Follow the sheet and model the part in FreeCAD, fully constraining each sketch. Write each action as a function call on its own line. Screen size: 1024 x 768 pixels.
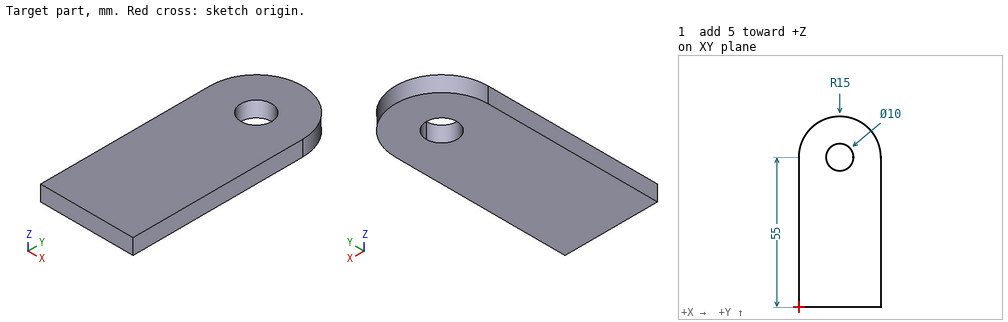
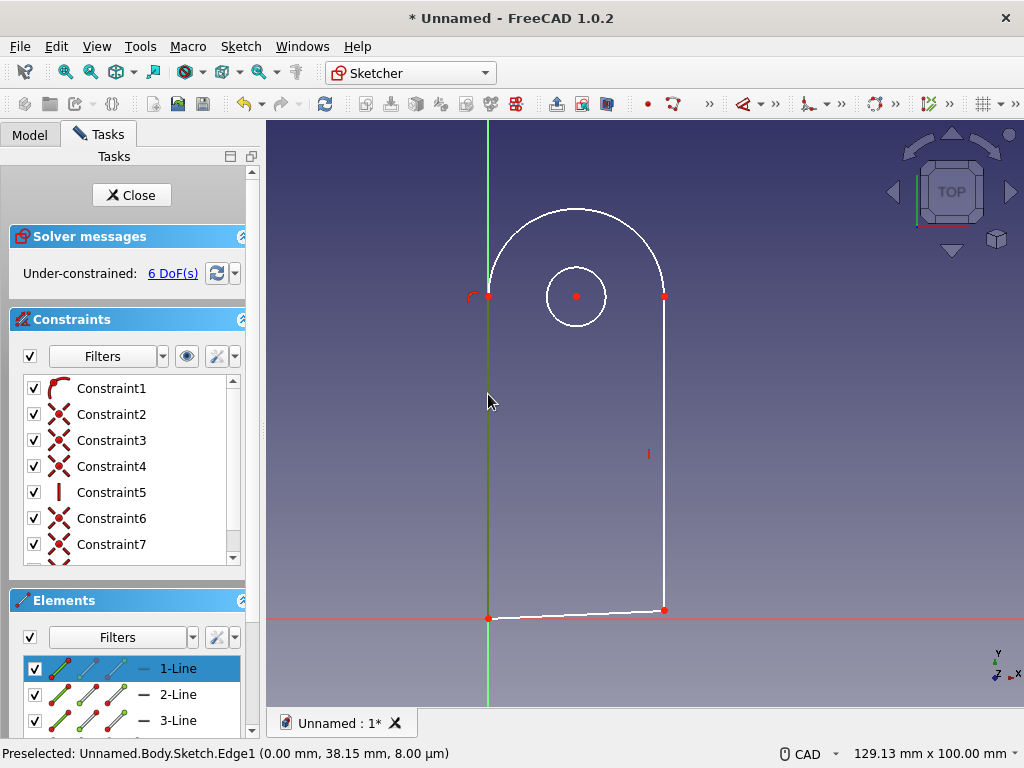
click(628, 226)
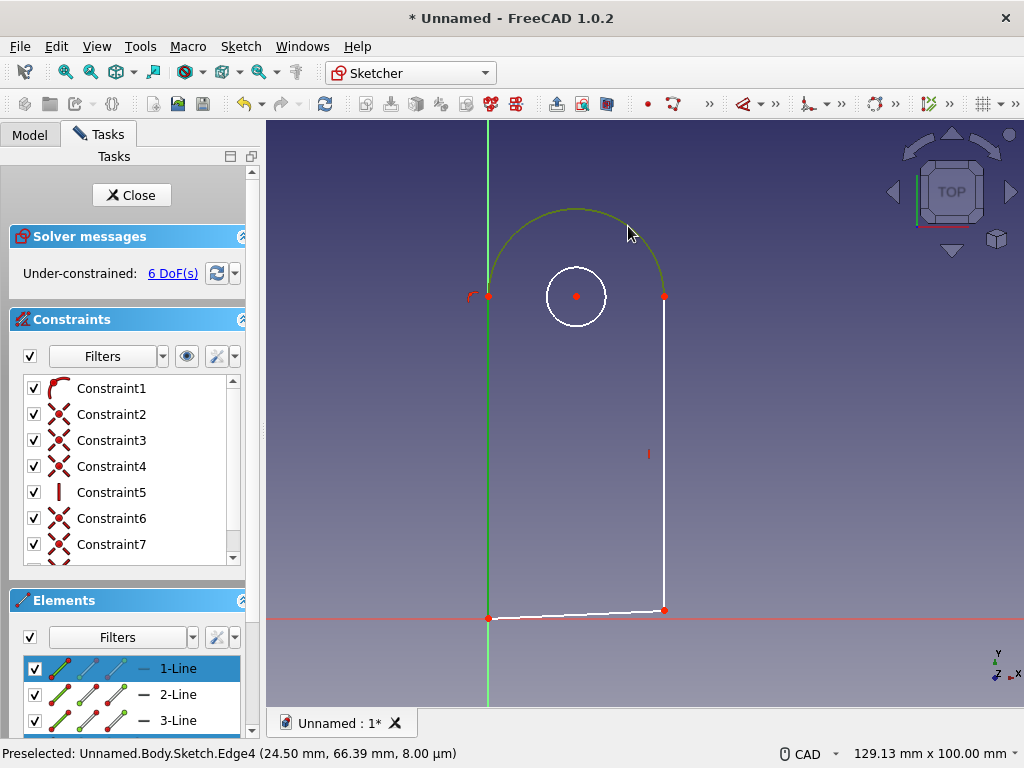
key(t)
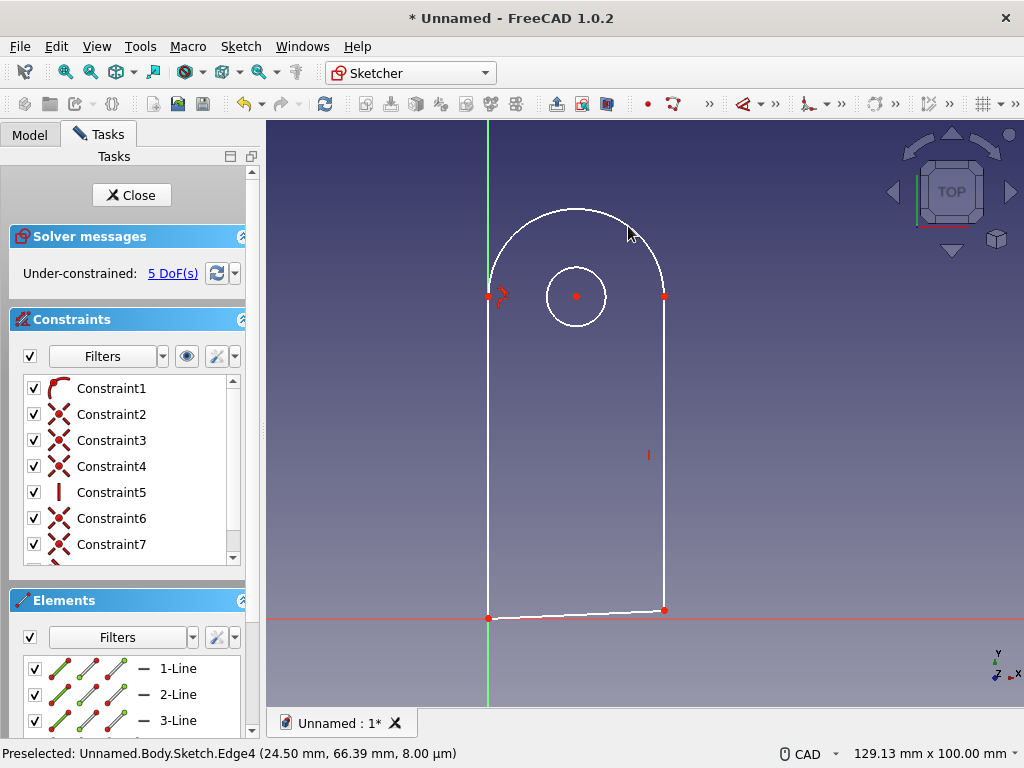
click(664, 517)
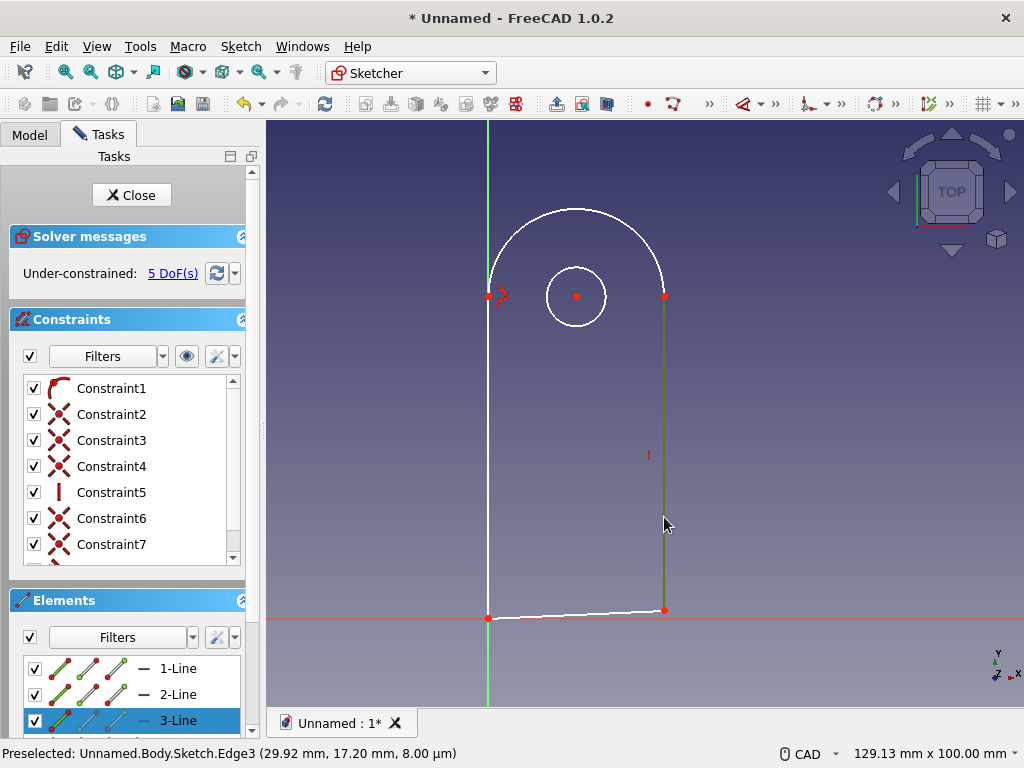
click(628, 226)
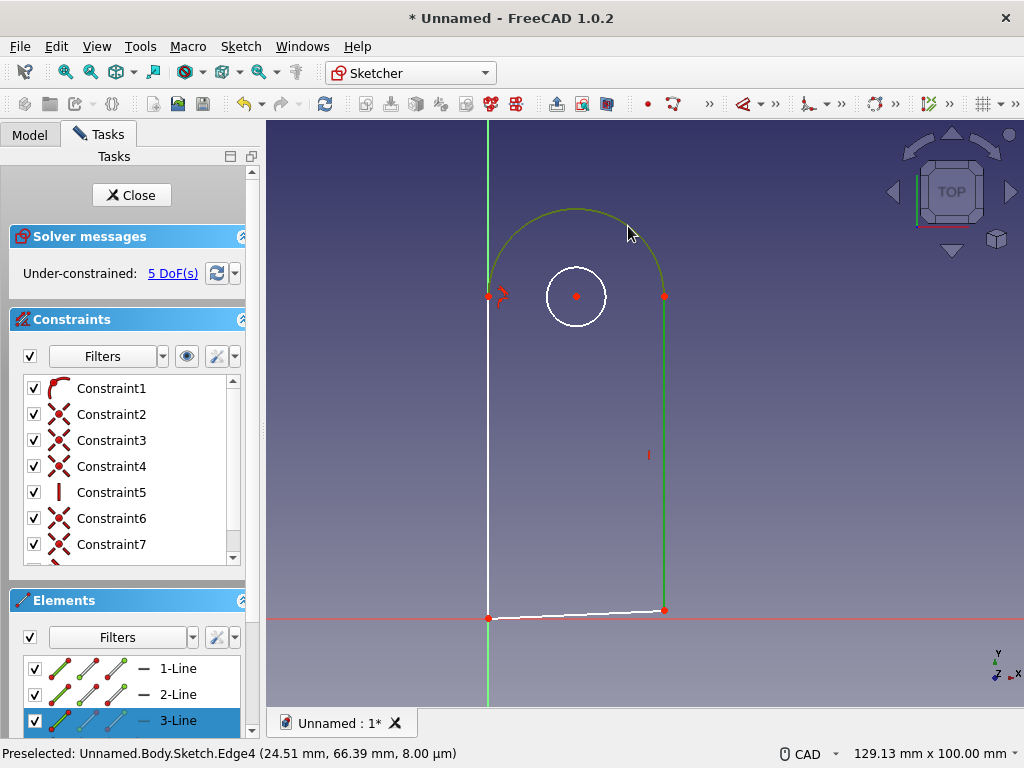
key(t)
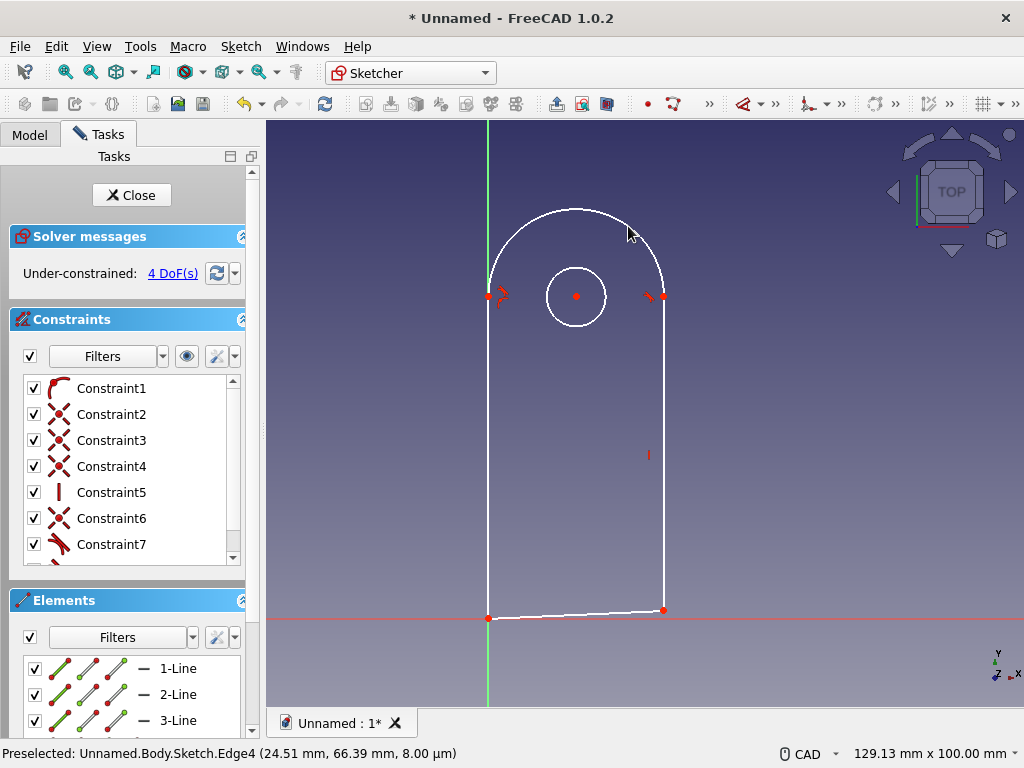
click(541, 617)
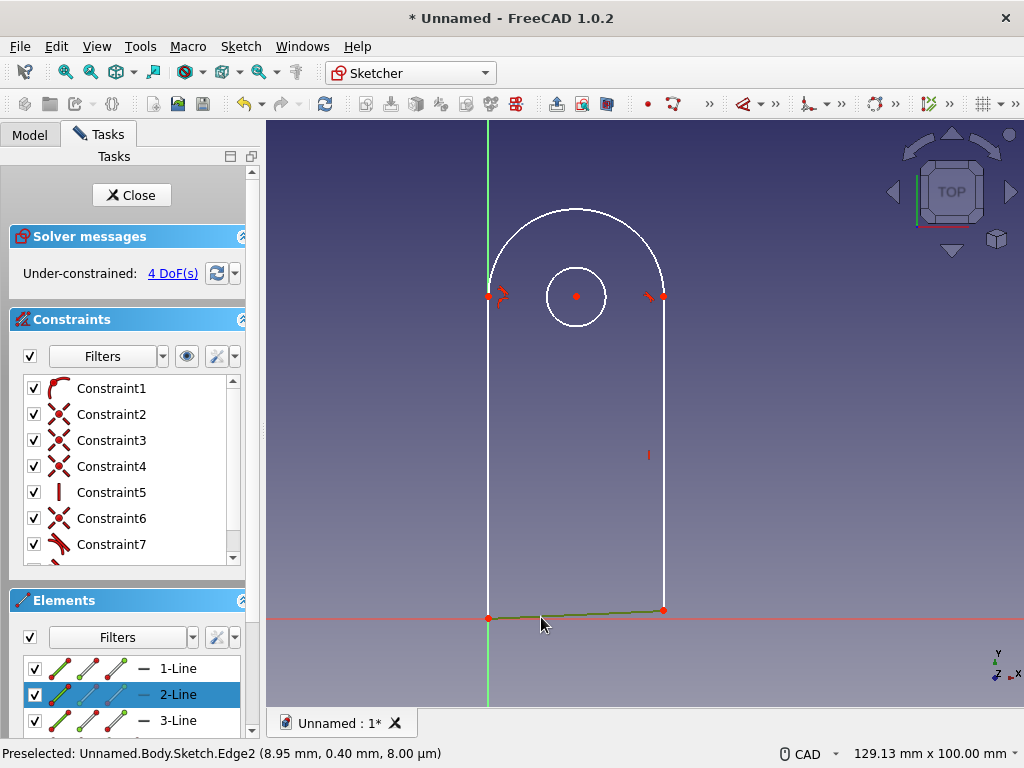
key(h)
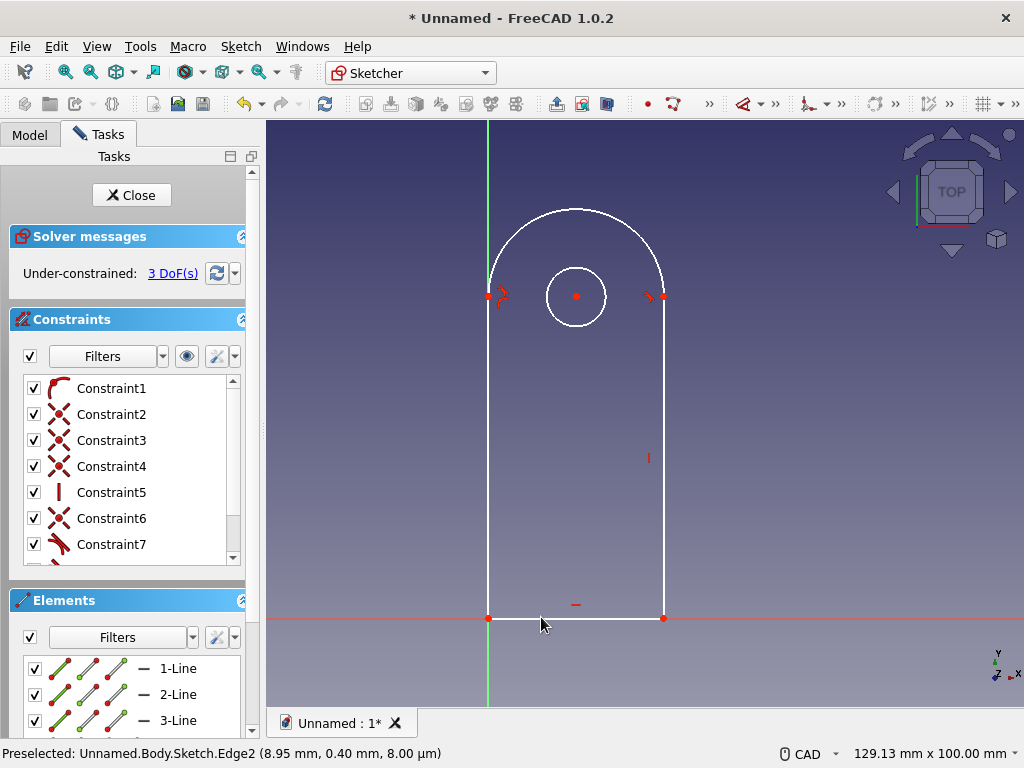
click(742, 104)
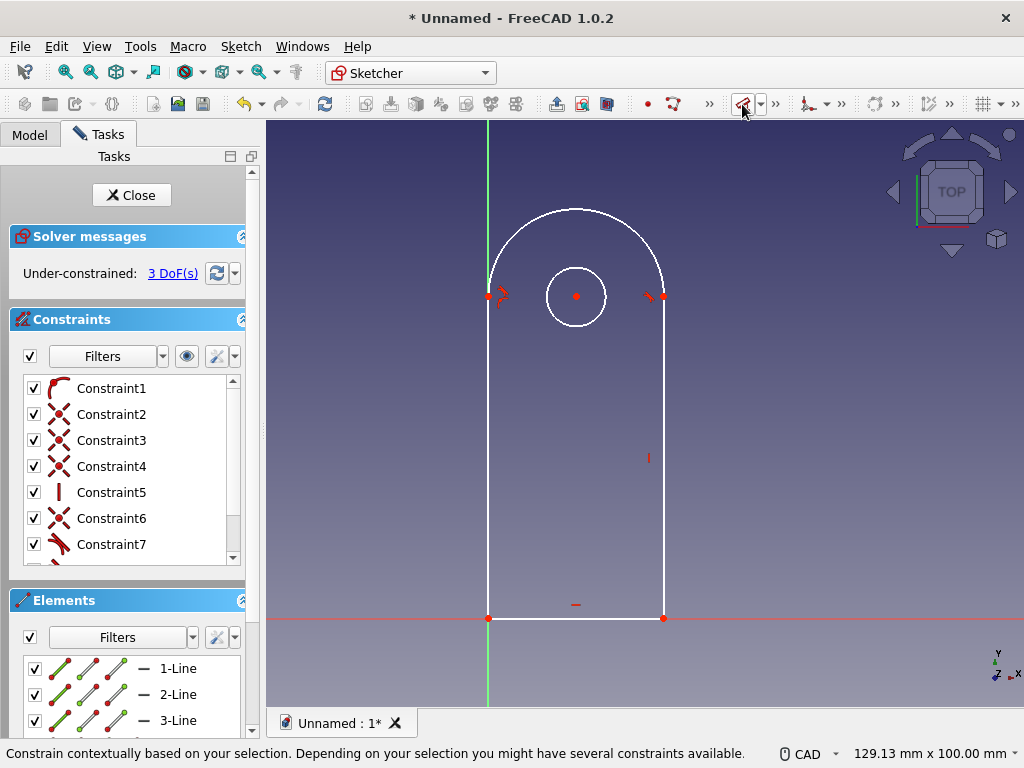
click(628, 226)
click(647, 200)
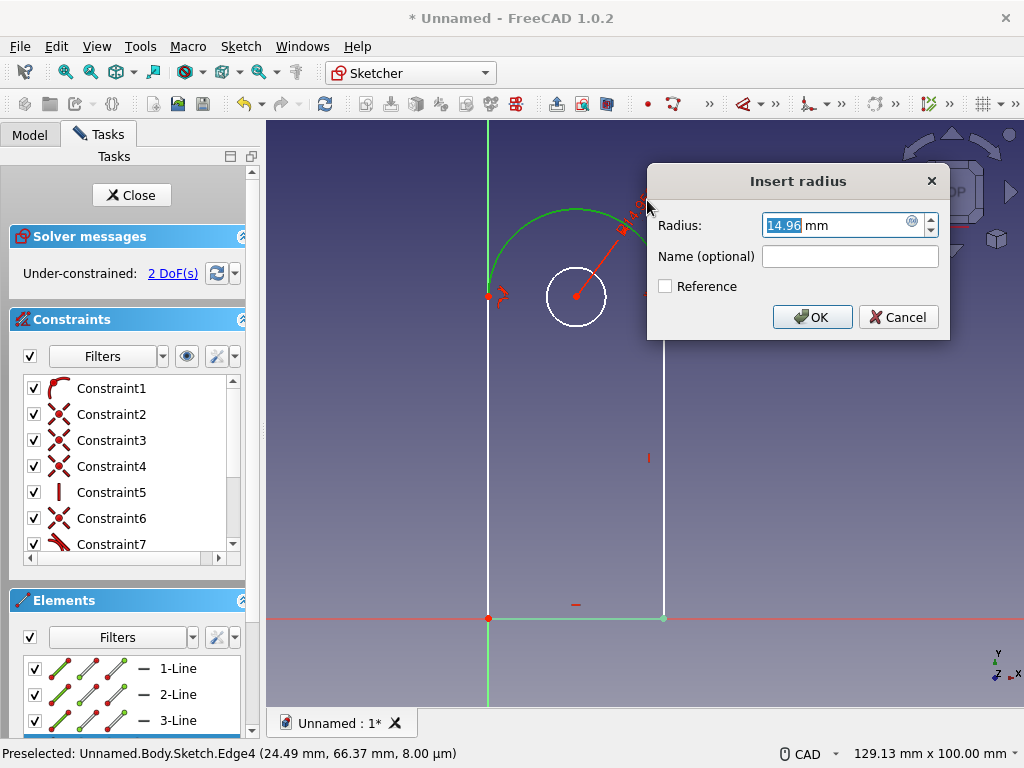
text(15)
key(Return)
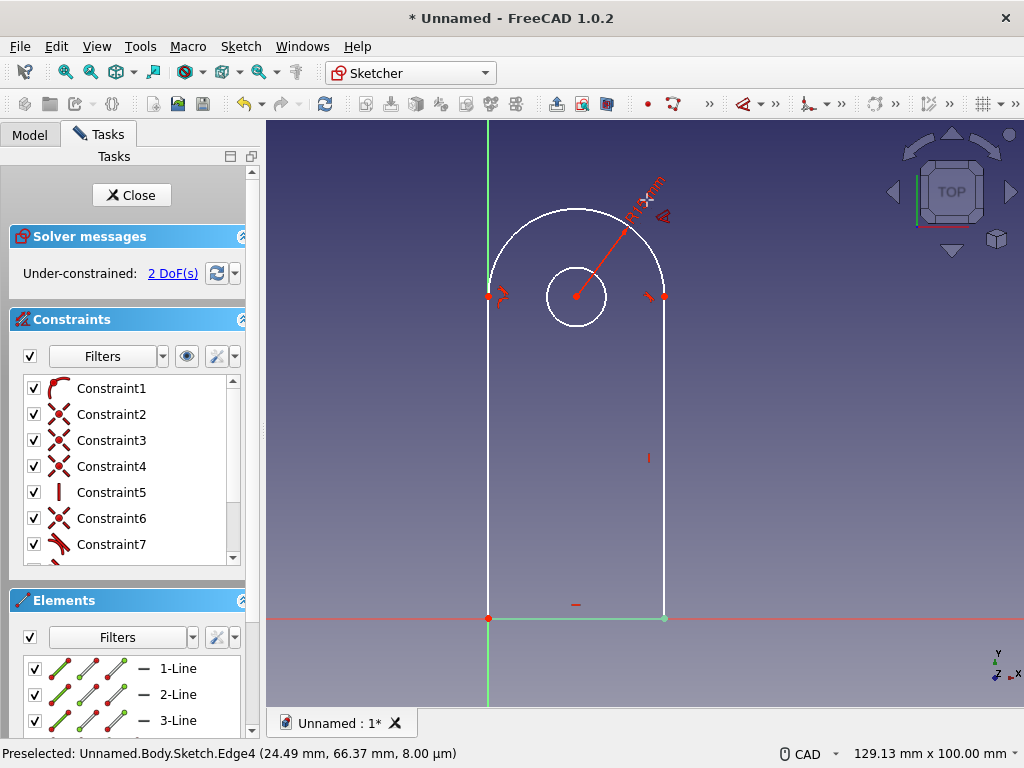
click(597, 276)
click(619, 253)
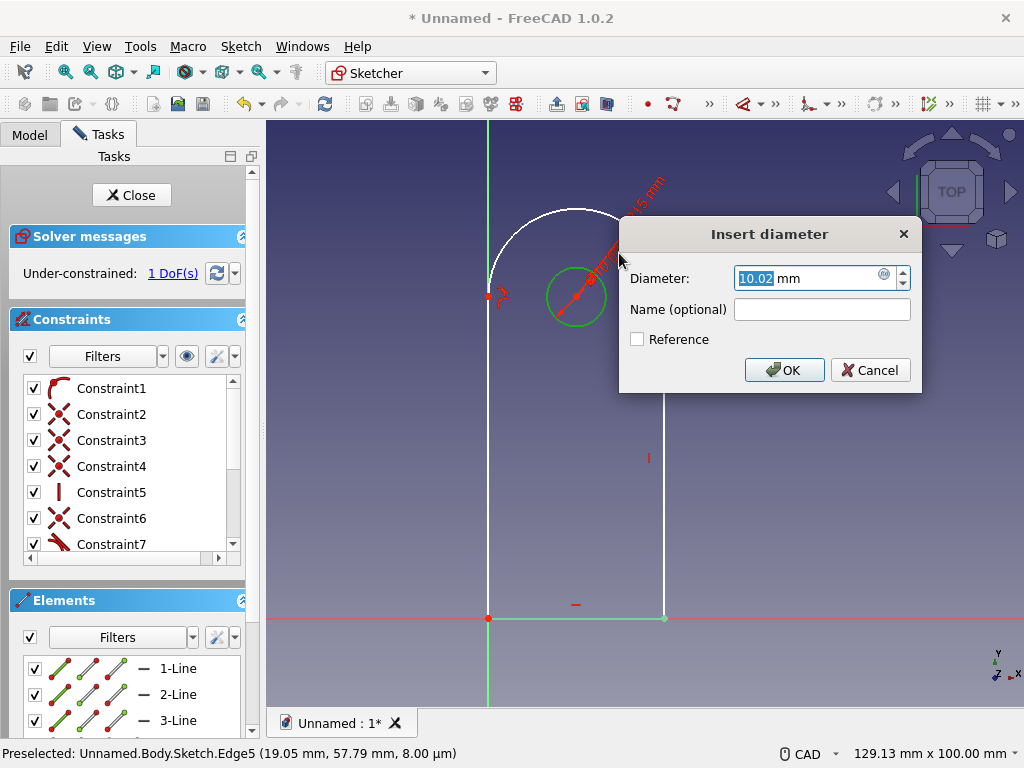
text(10)
key(Return)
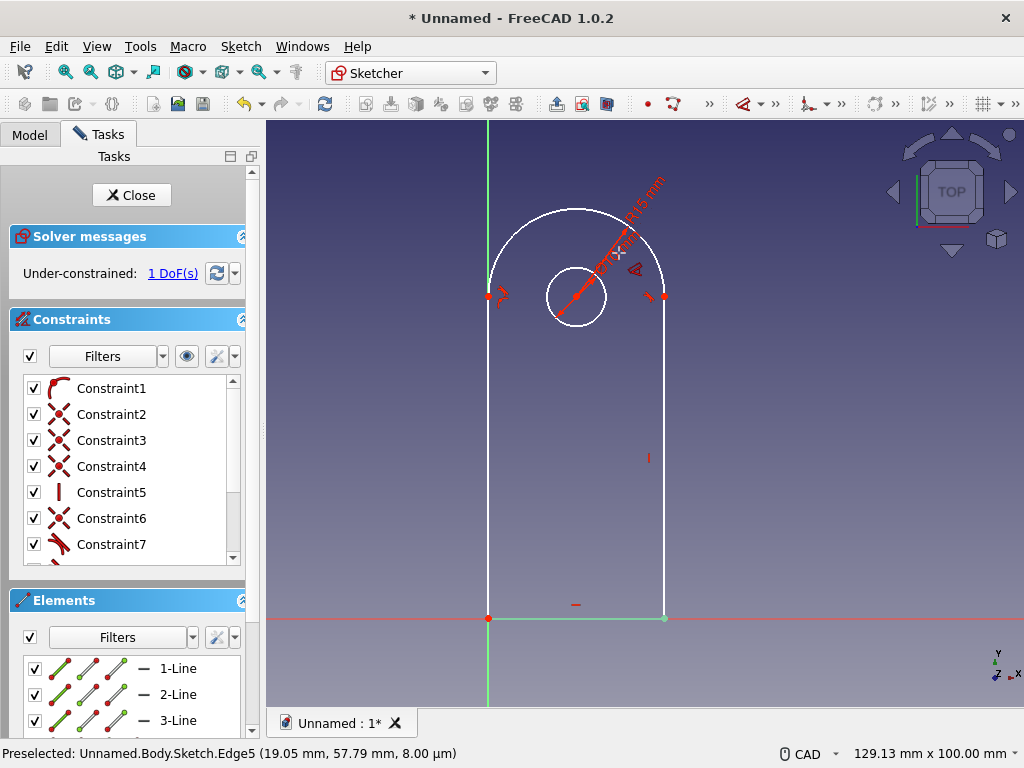
click(488, 394)
click(454, 458)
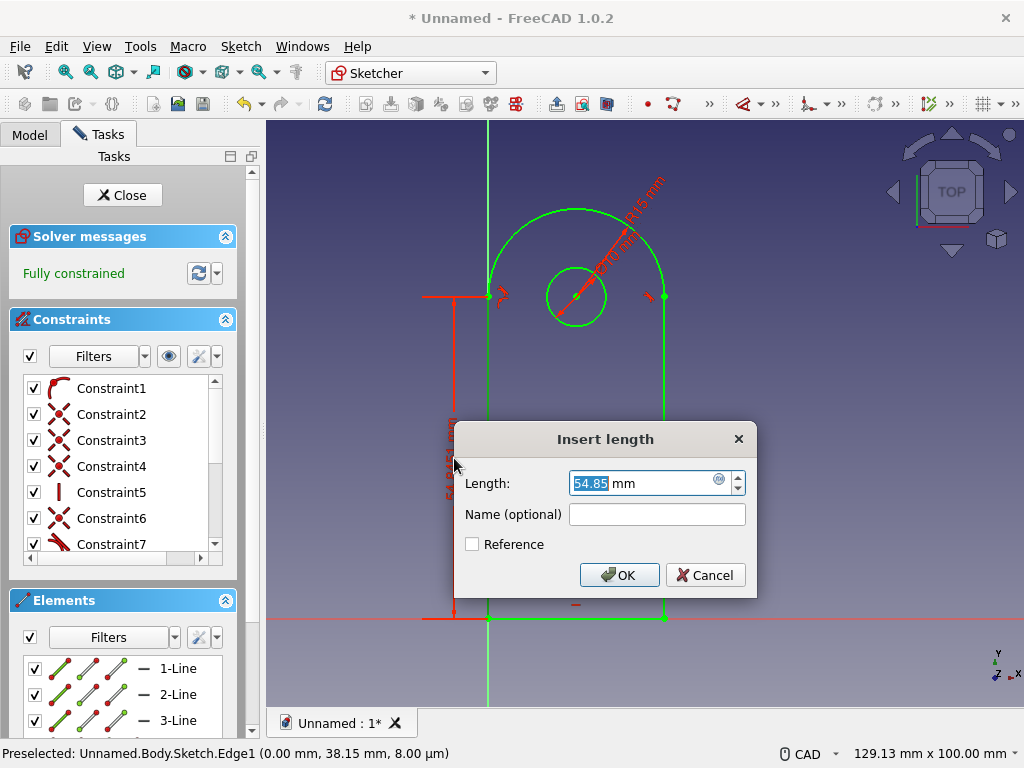
text(55)
key(Return)
key(Escape)